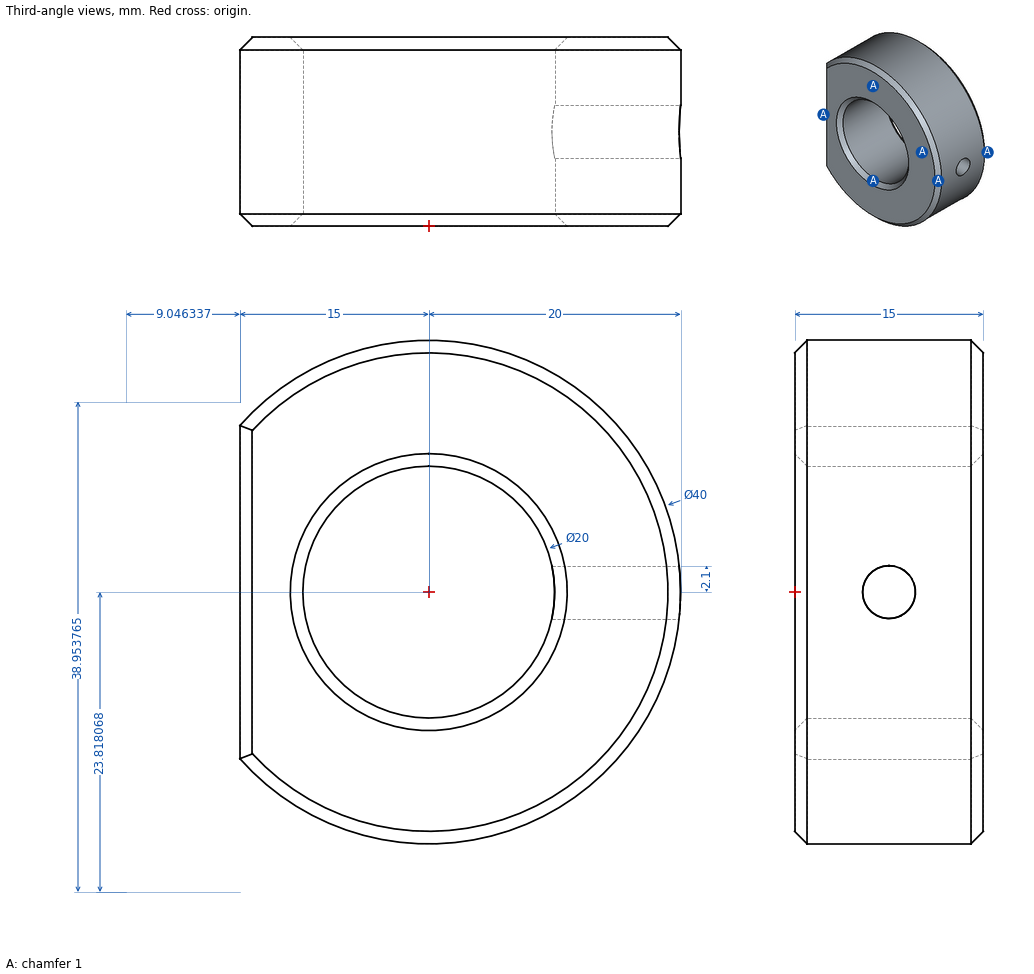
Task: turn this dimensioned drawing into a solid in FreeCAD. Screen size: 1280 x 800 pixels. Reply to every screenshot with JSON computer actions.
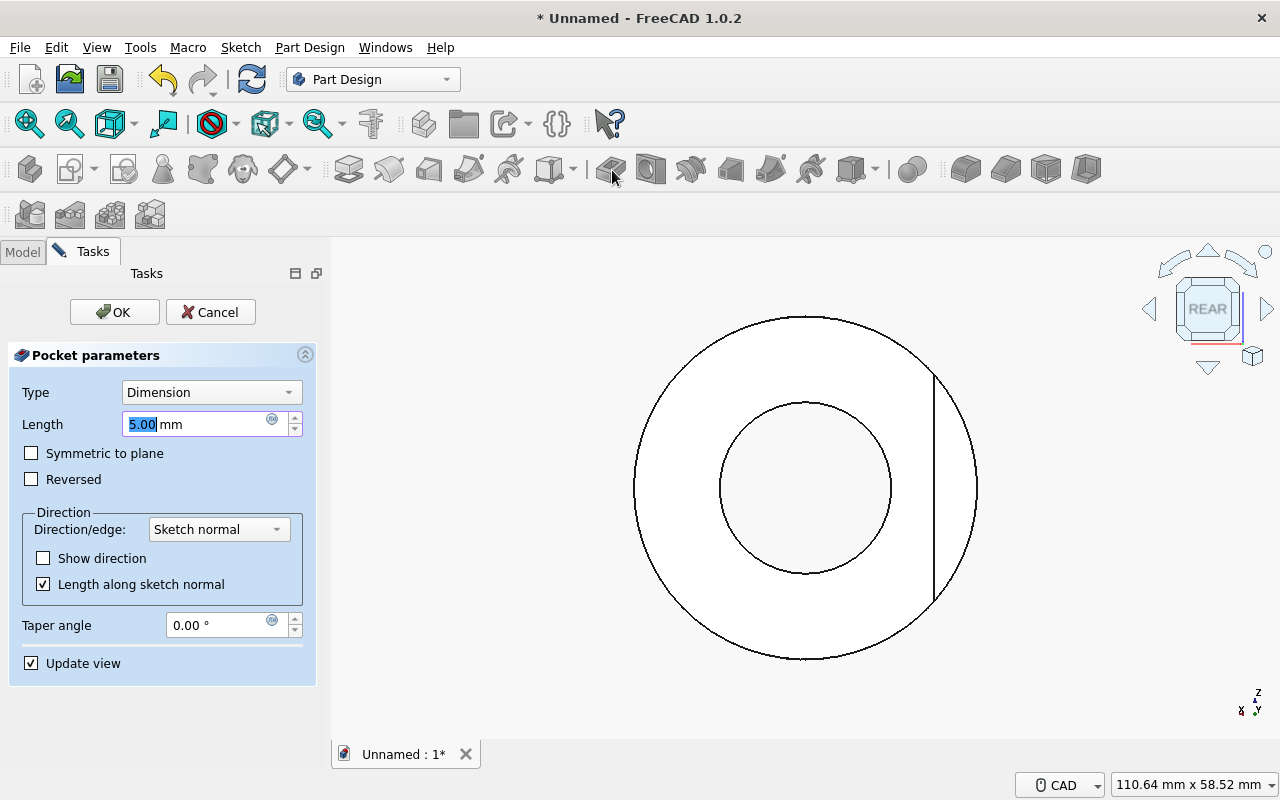
{"action": "left_click", "coordinate": [212, 392]}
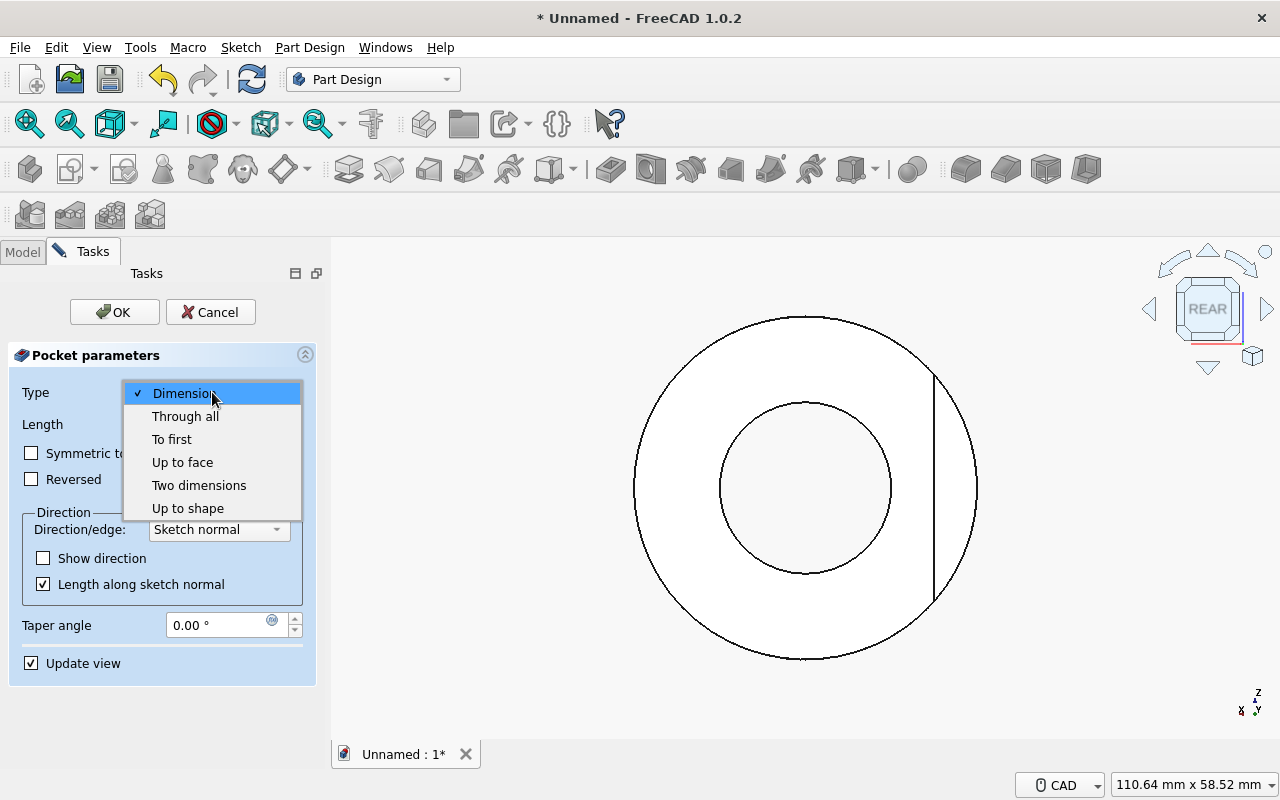
{"action": "left_click", "coordinate": [212, 416]}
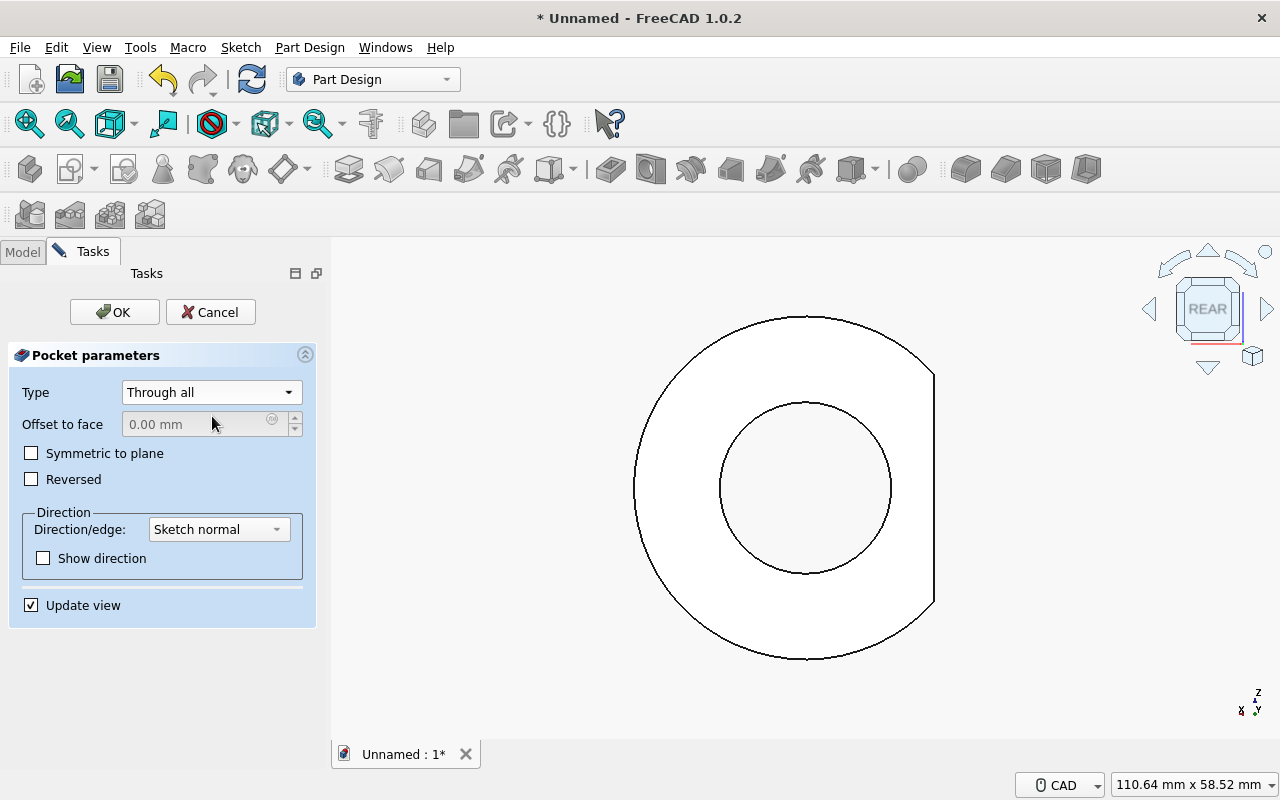
{"action": "left_click", "coordinate": [115, 312]}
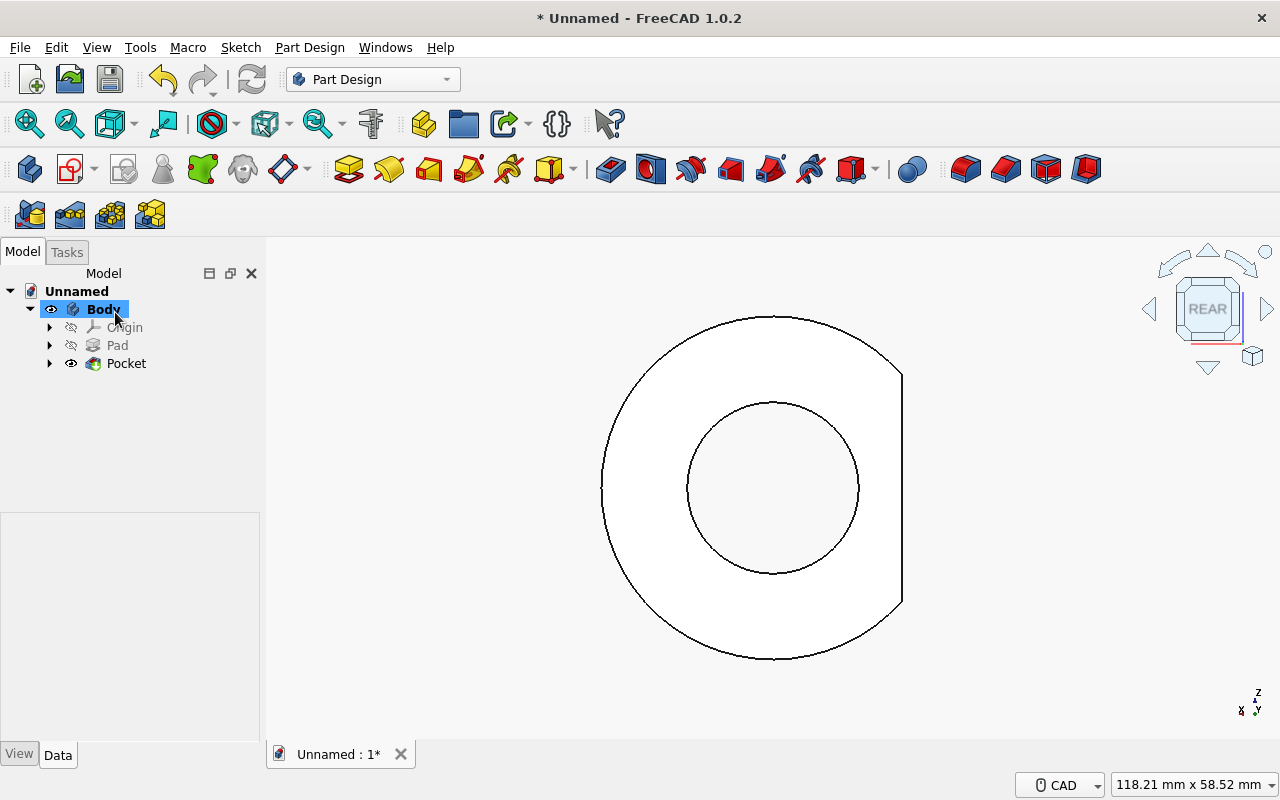
{"action": "left_click", "coordinate": [902, 487]}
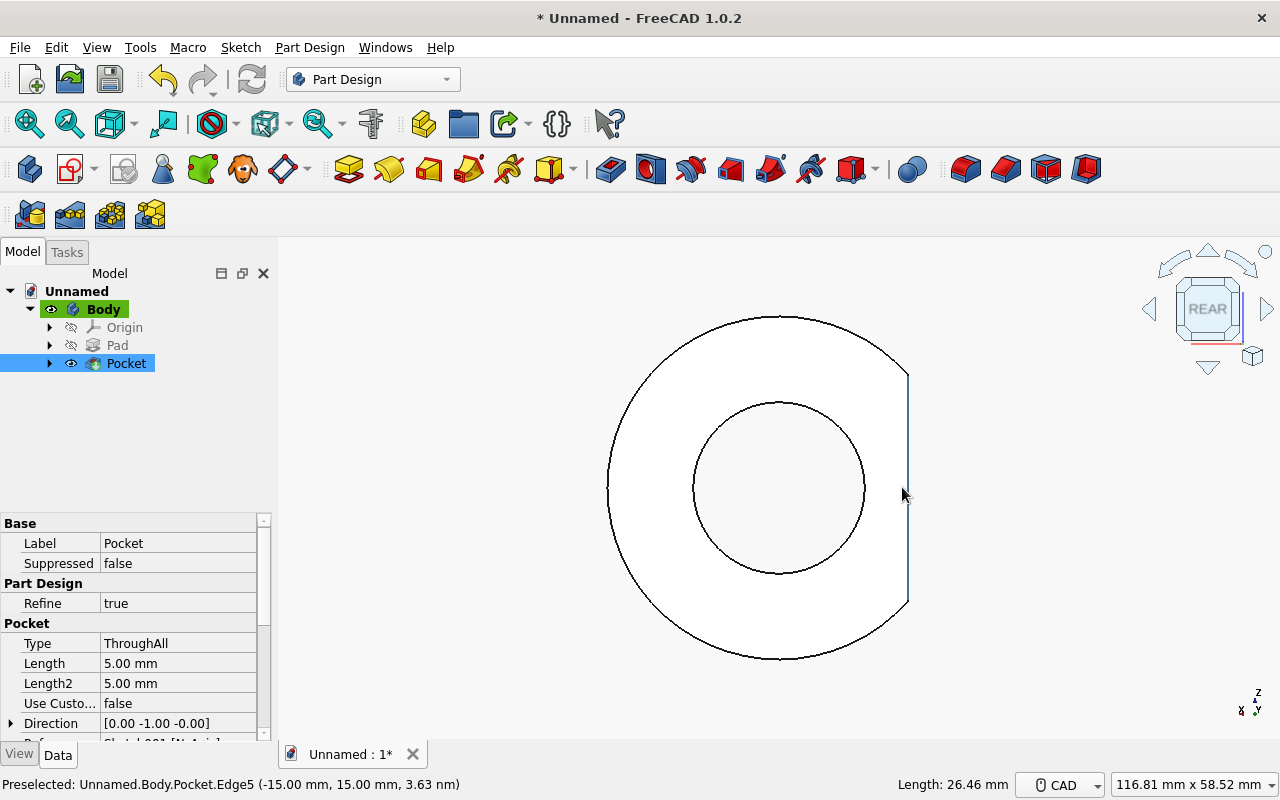
{"action": "left_click", "coordinate": [848, 437], "text": "ctrl"}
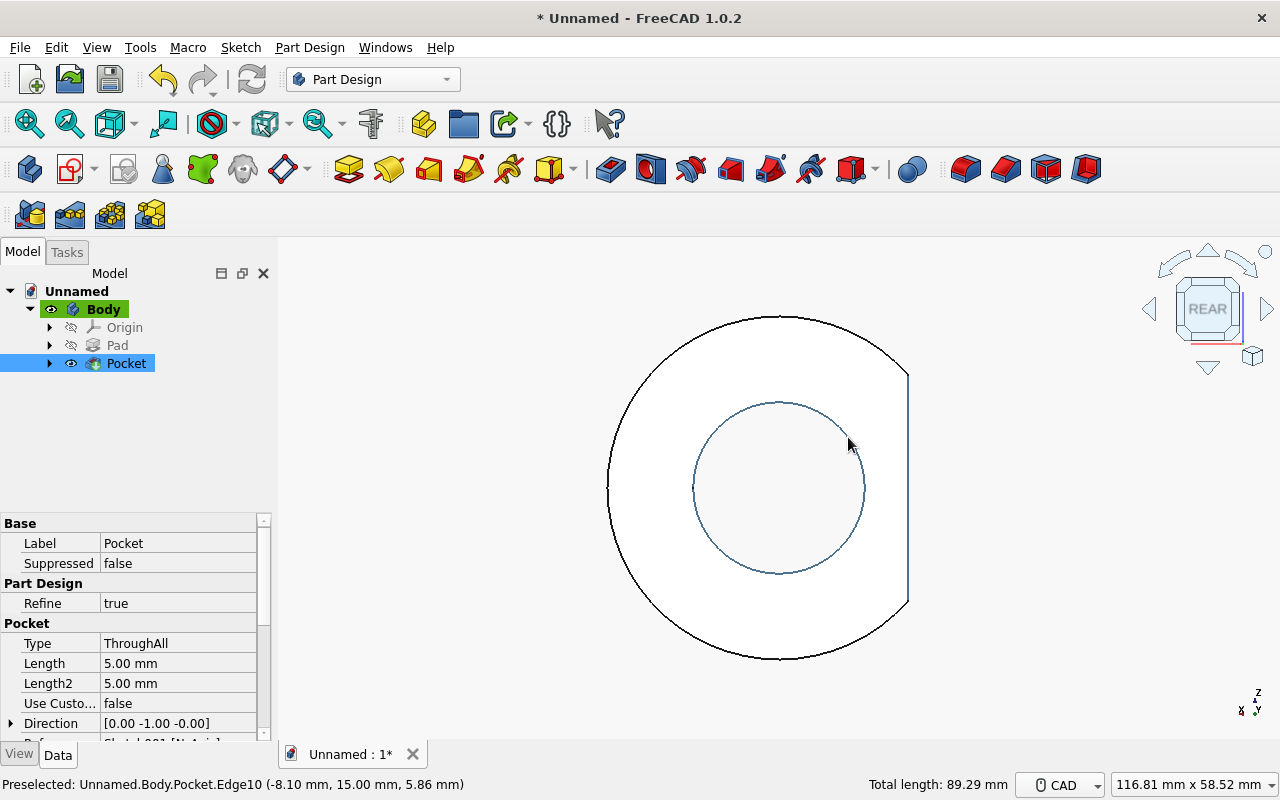
{"action": "key", "text": "0"}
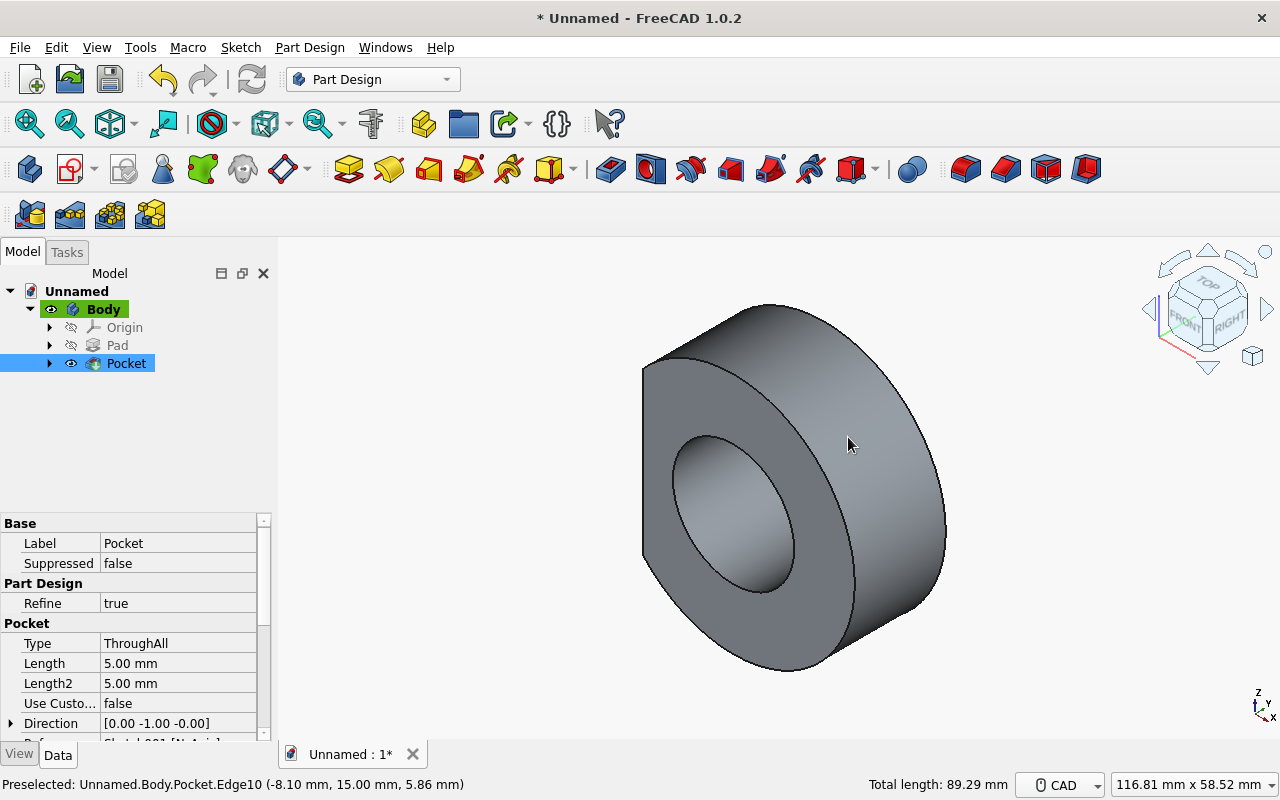
{"action": "left_click", "coordinate": [776, 407], "text": "ctrl"}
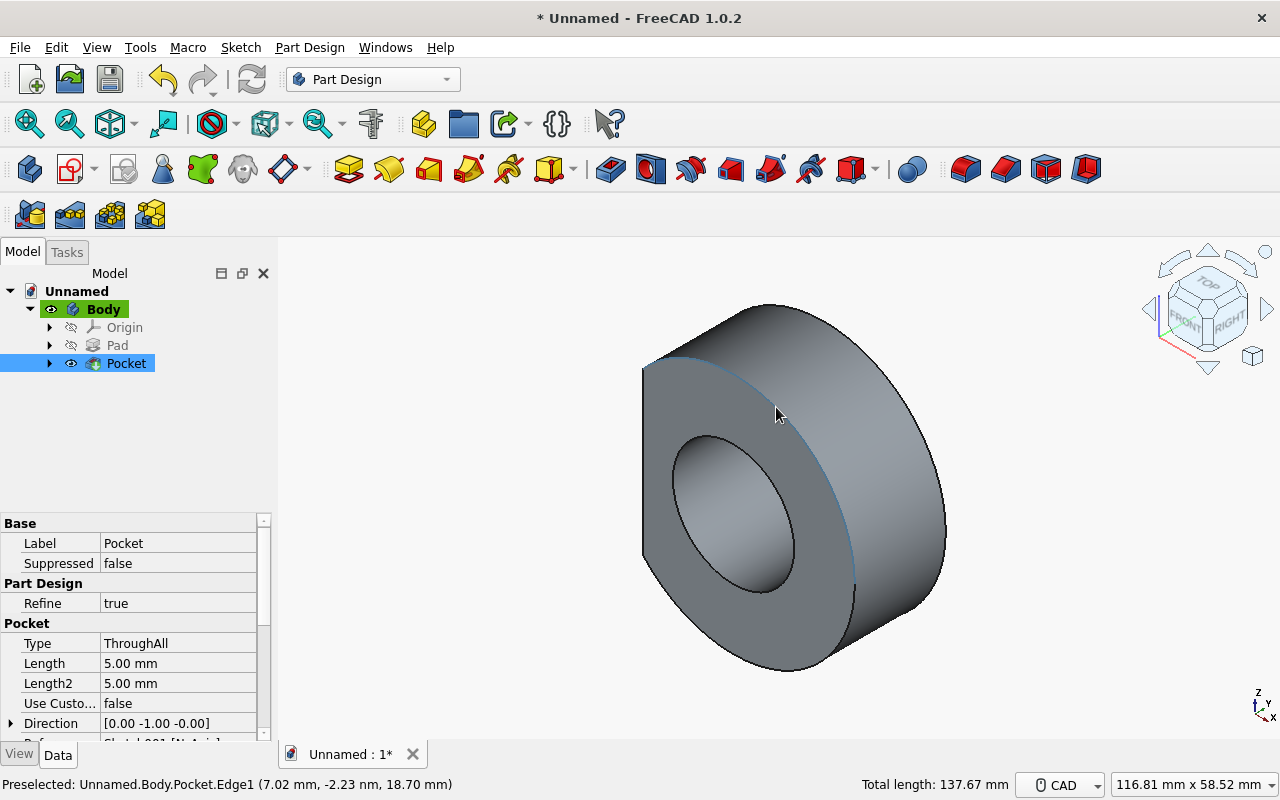
{"action": "left_click", "coordinate": [673, 478], "text": "ctrl"}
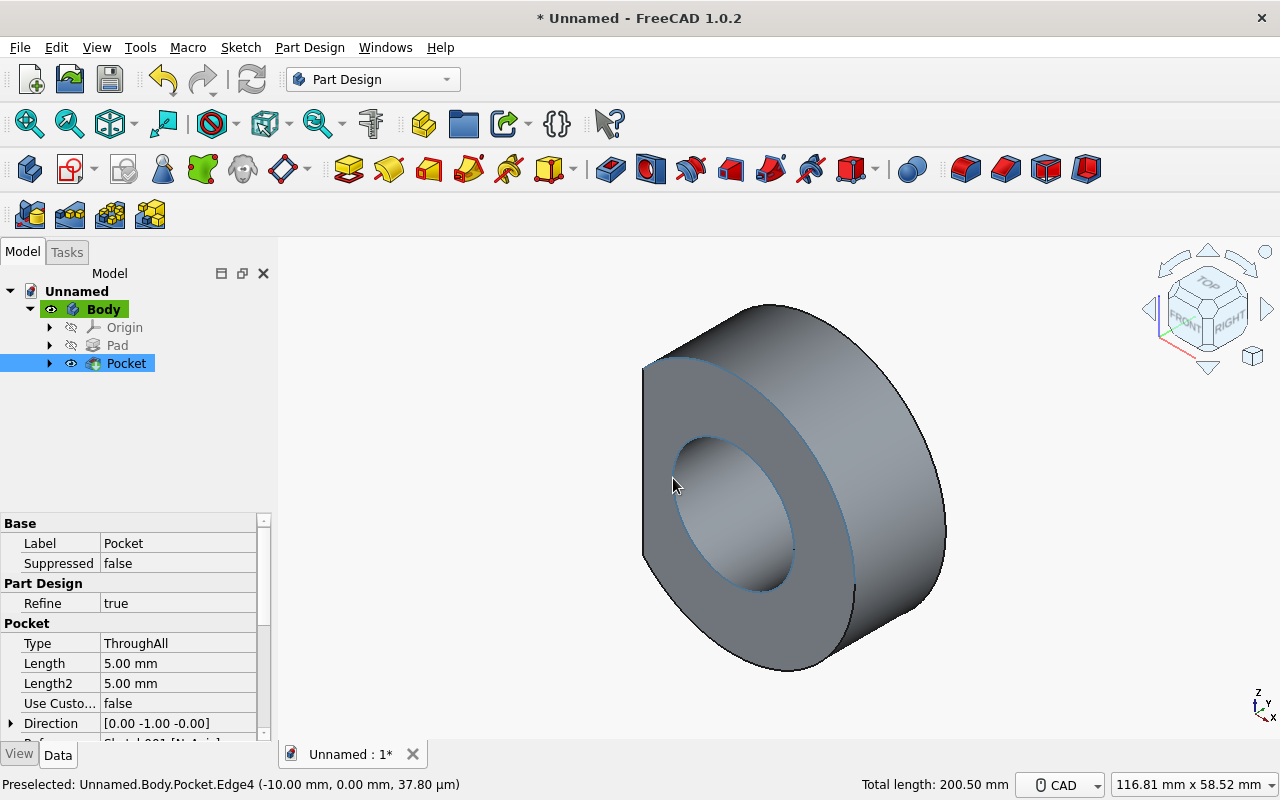
{"action": "key", "text": "2"}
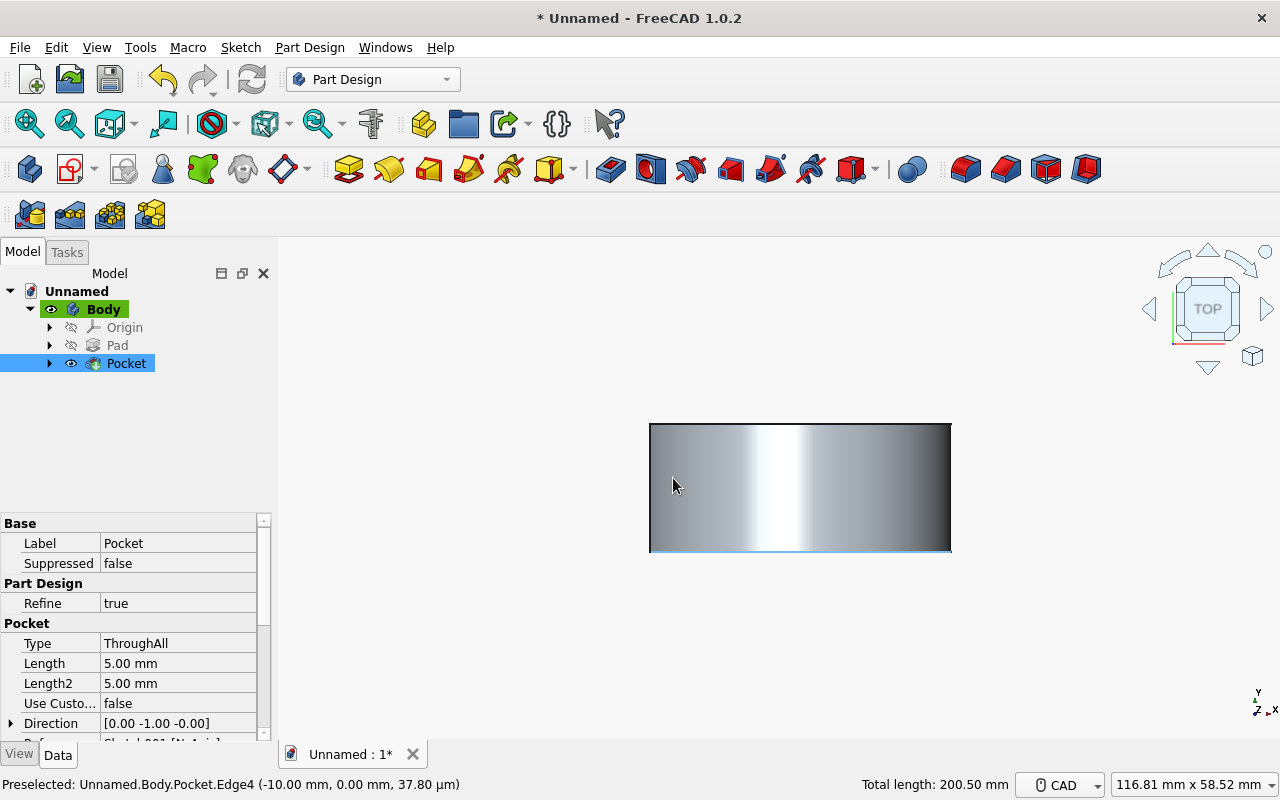
{"action": "left_click", "coordinate": [30, 124]}